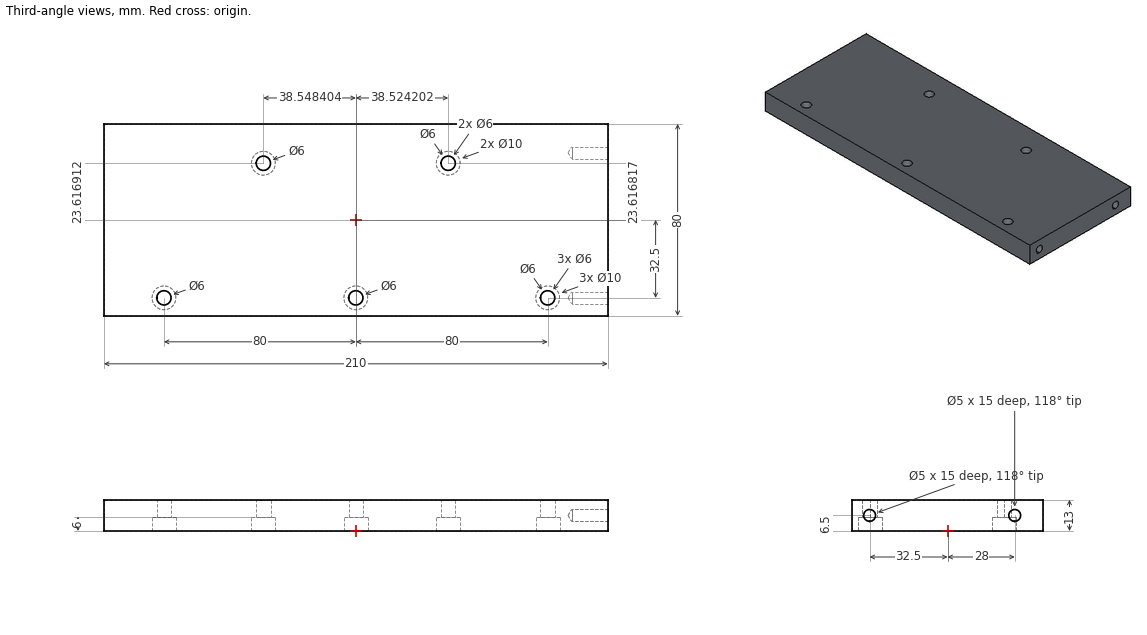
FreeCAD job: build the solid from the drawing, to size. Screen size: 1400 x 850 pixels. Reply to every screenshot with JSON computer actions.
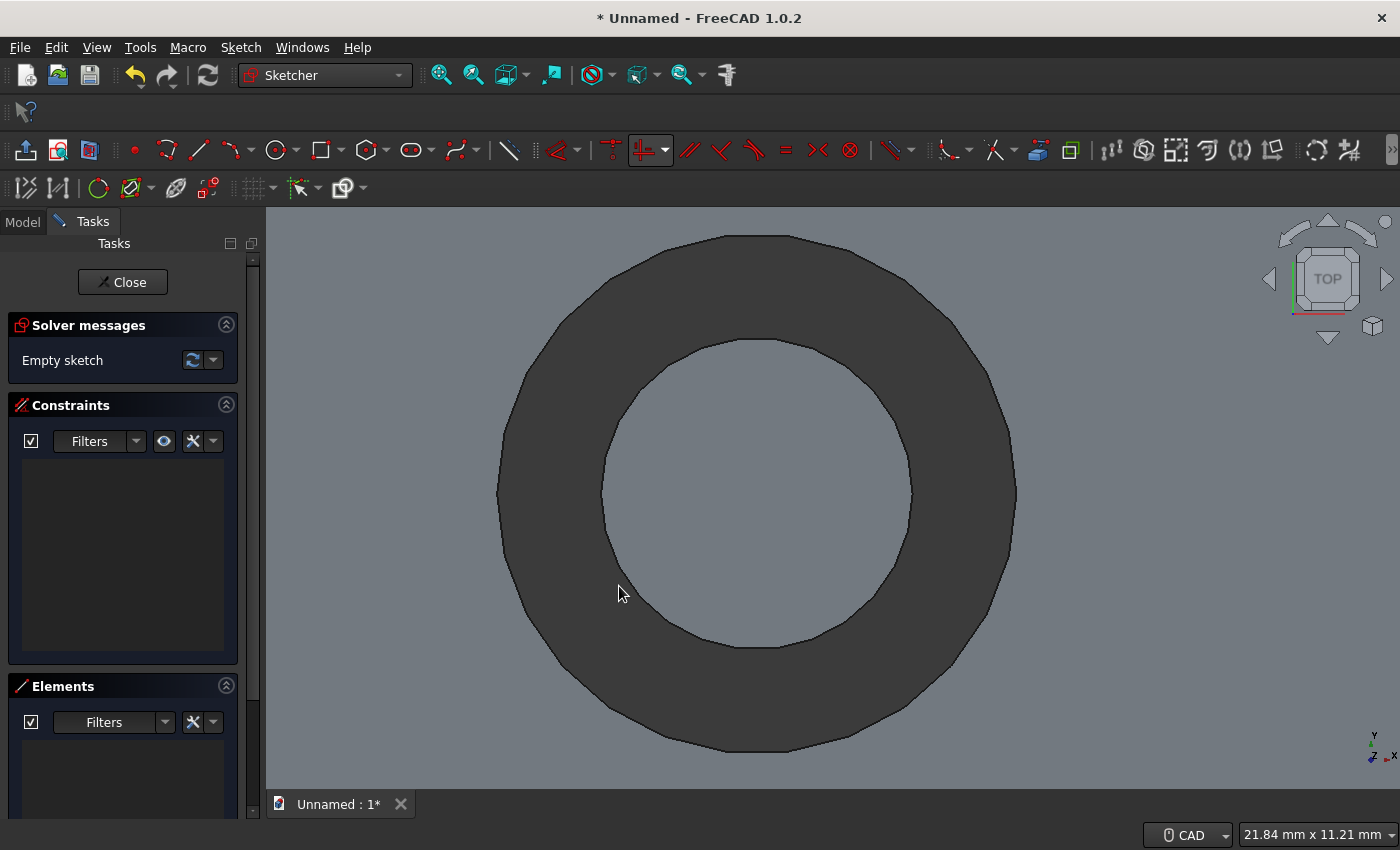
{"action": "key", "text": "g c"}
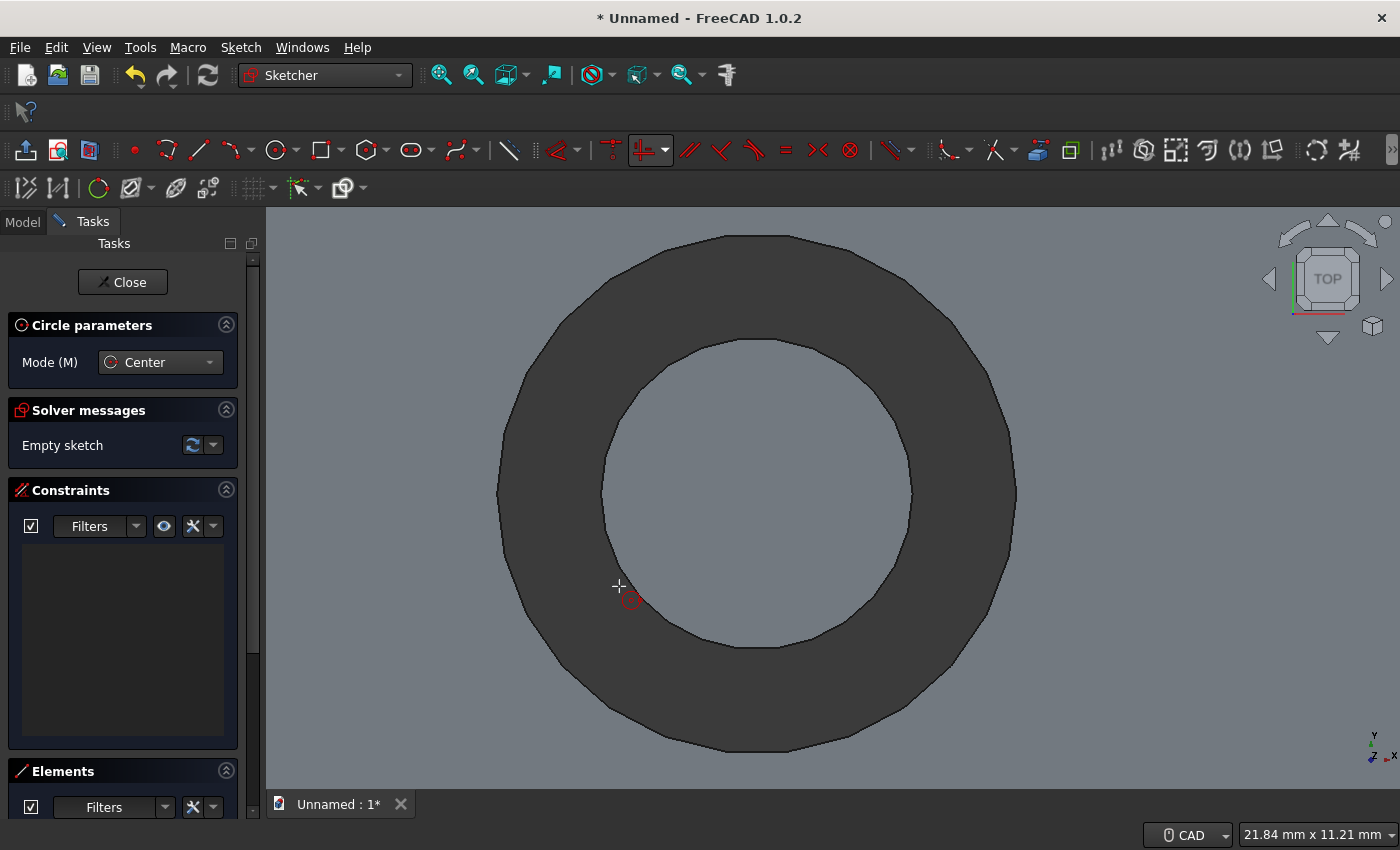
{"action": "left_click", "coordinate": [757, 494]}
{"action": "left_click", "coordinate": [867, 384]}
{"action": "key", "text": "Escape"}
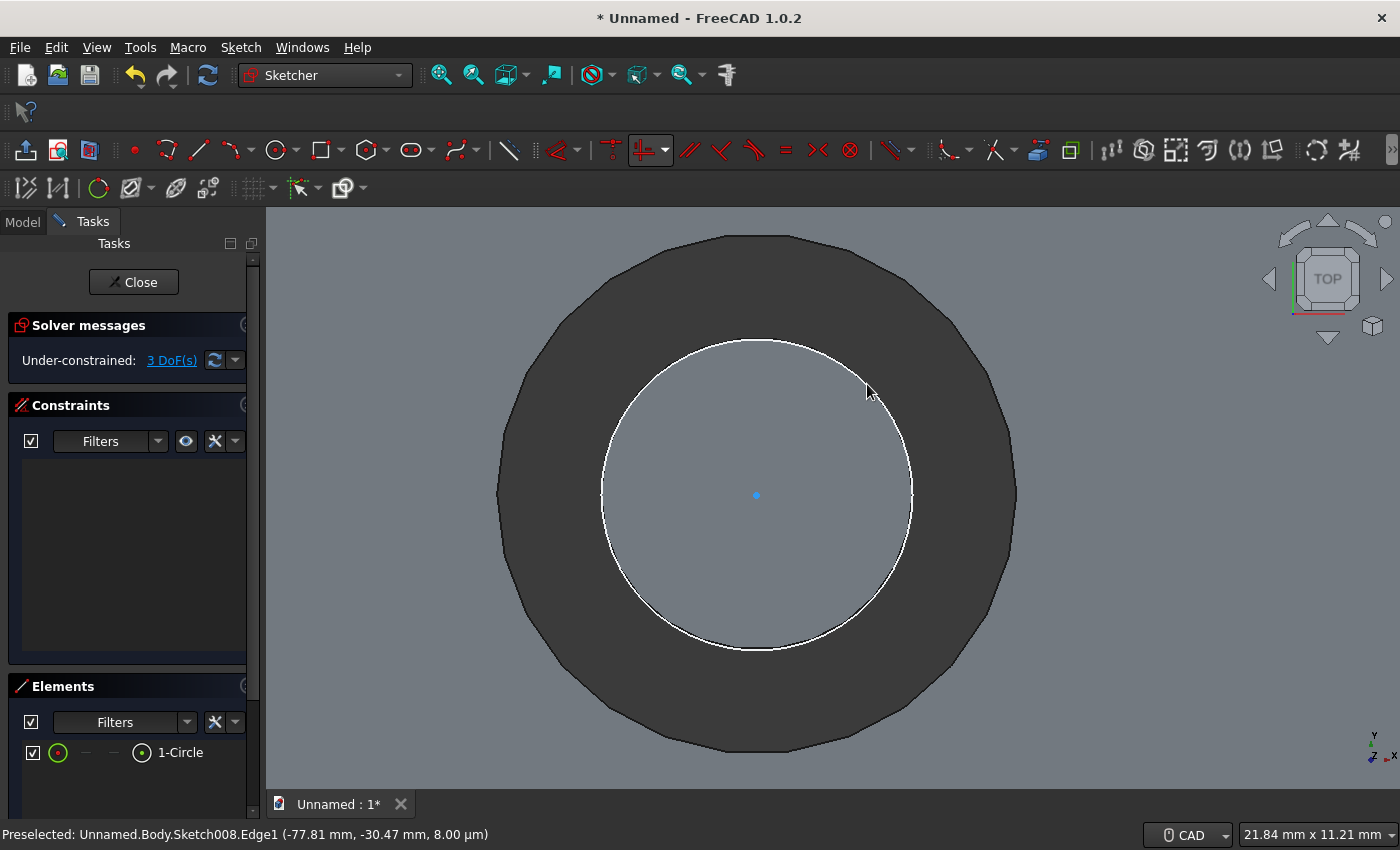
{"action": "left_click", "coordinate": [556, 150]}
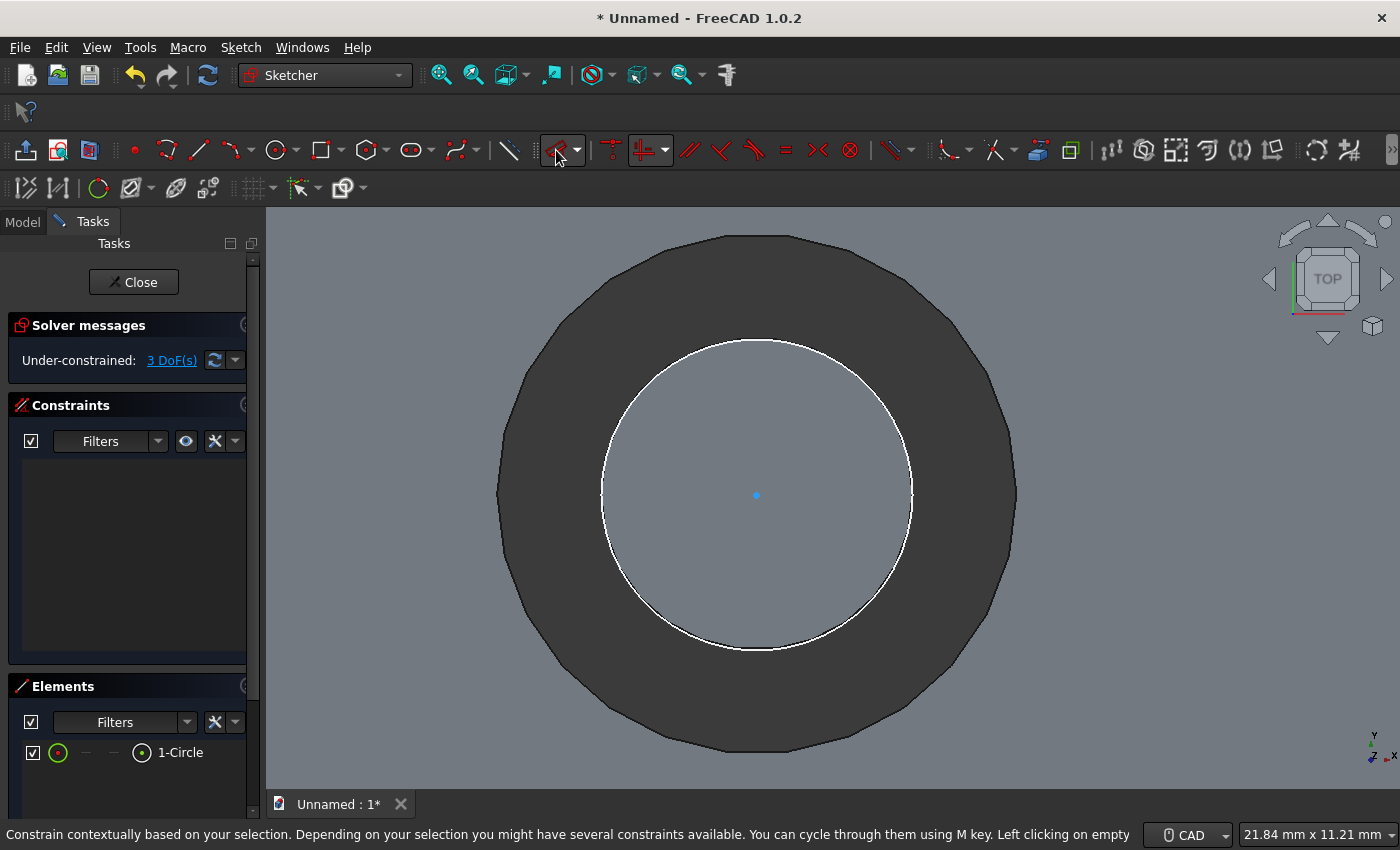
{"action": "left_click", "coordinate": [867, 385]}
{"action": "left_click", "coordinate": [890, 362]}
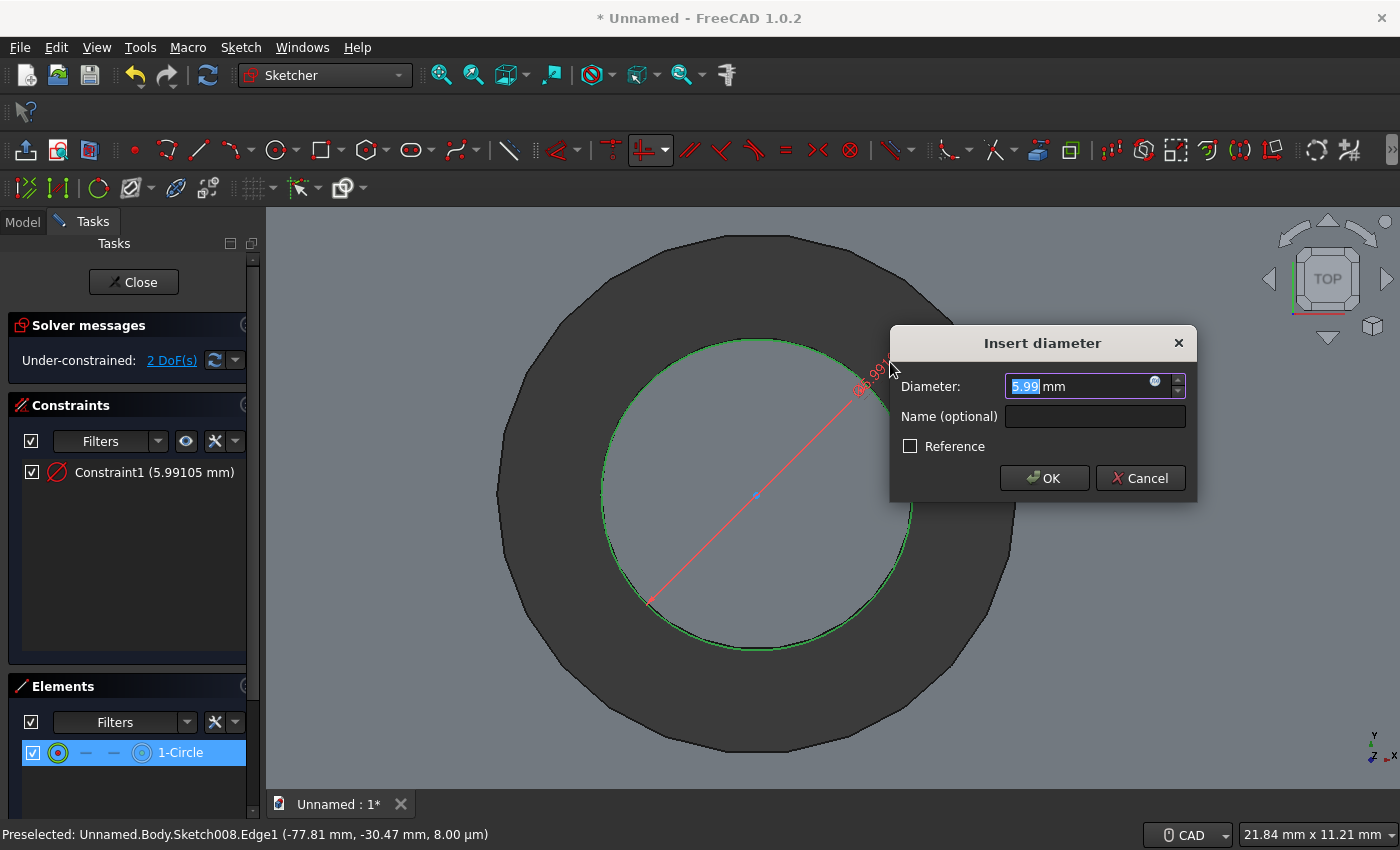
{"action": "type", "text": "6"}
{"action": "key", "text": "Return"}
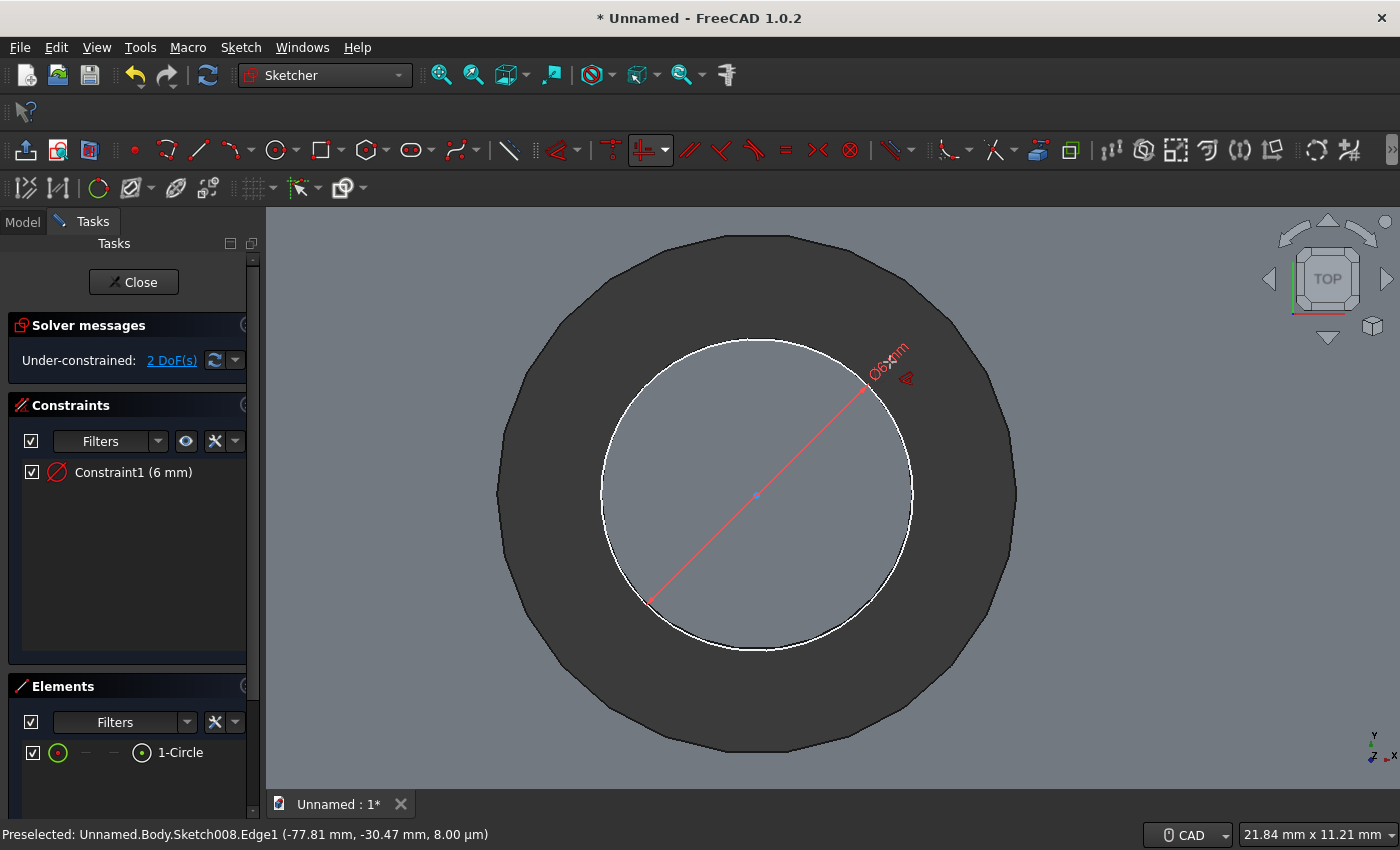
{"action": "left_click", "coordinate": [757, 495]}
{"action": "left_click", "coordinate": [996, 529]}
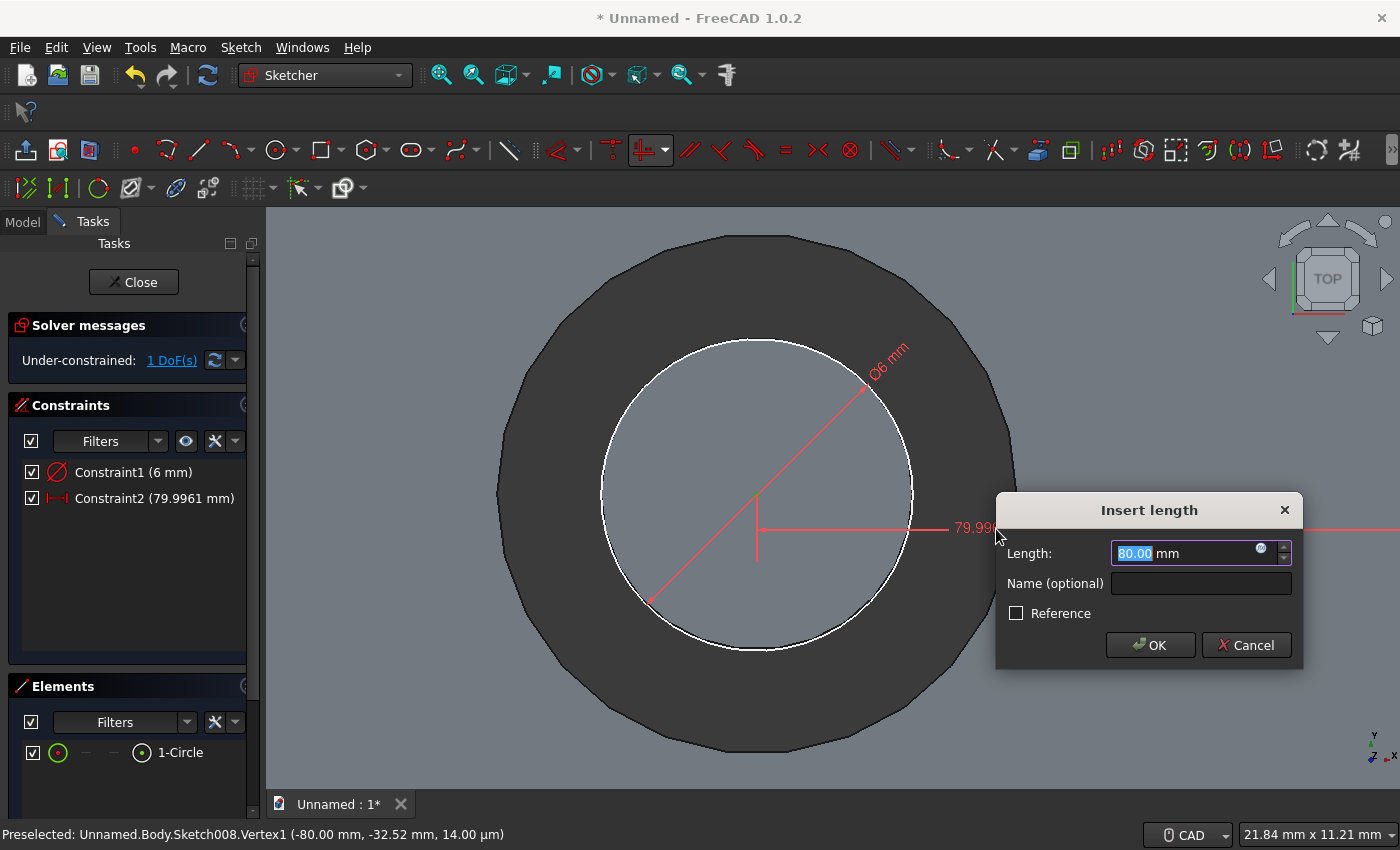
{"action": "type", "text": "80"}
{"action": "key", "text": "Return"}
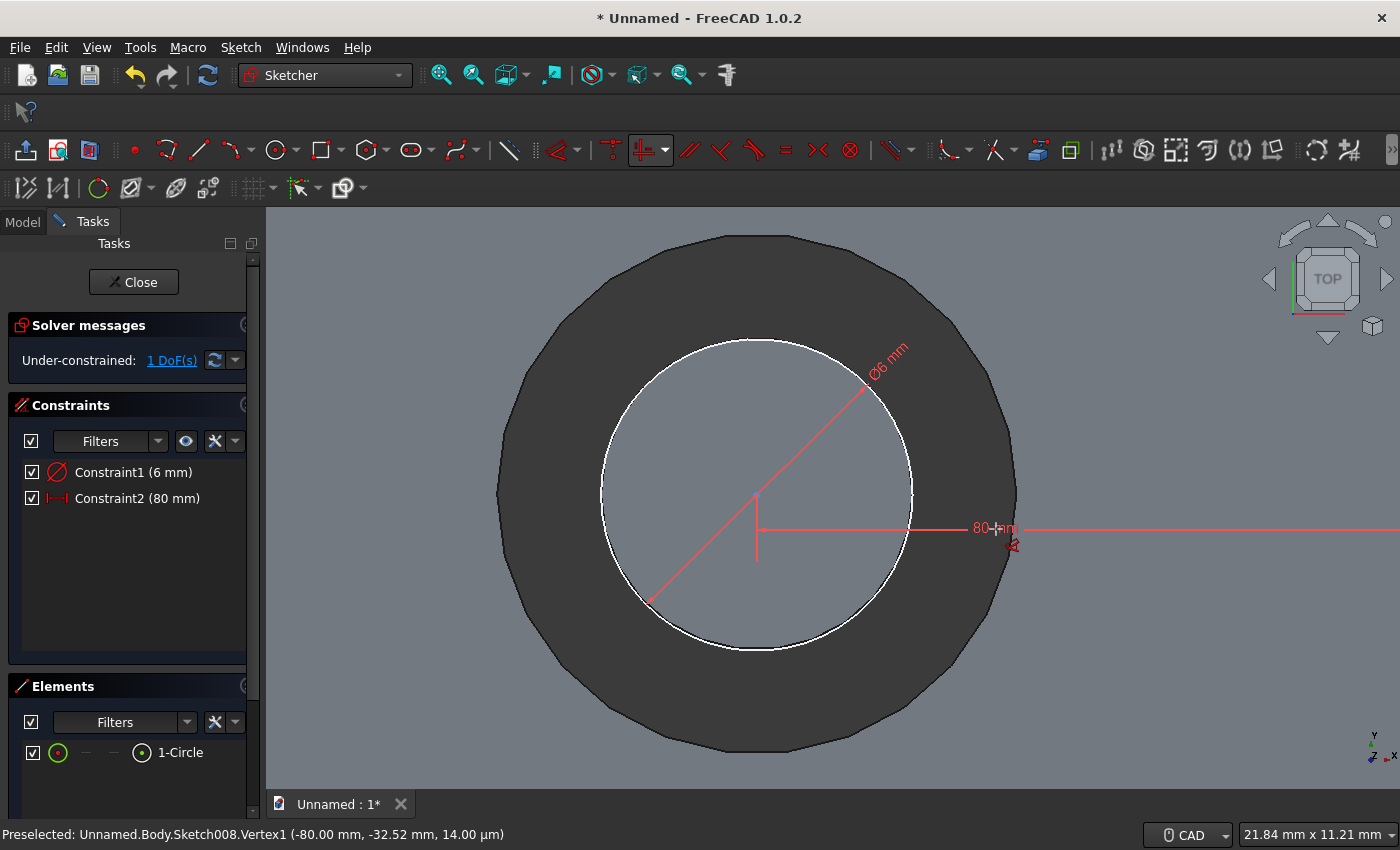
{"action": "left_click", "coordinate": [757, 495]}
{"action": "left_click", "coordinate": [723, 365]}